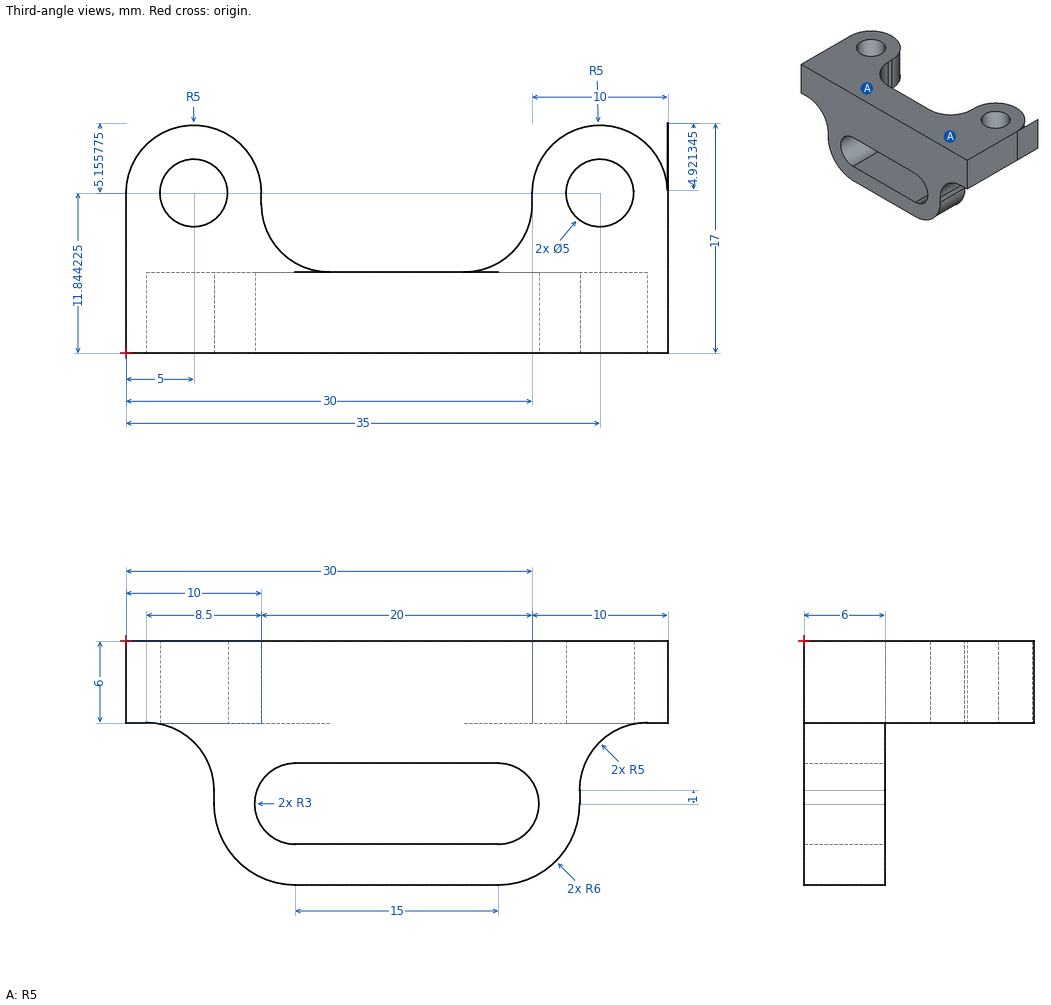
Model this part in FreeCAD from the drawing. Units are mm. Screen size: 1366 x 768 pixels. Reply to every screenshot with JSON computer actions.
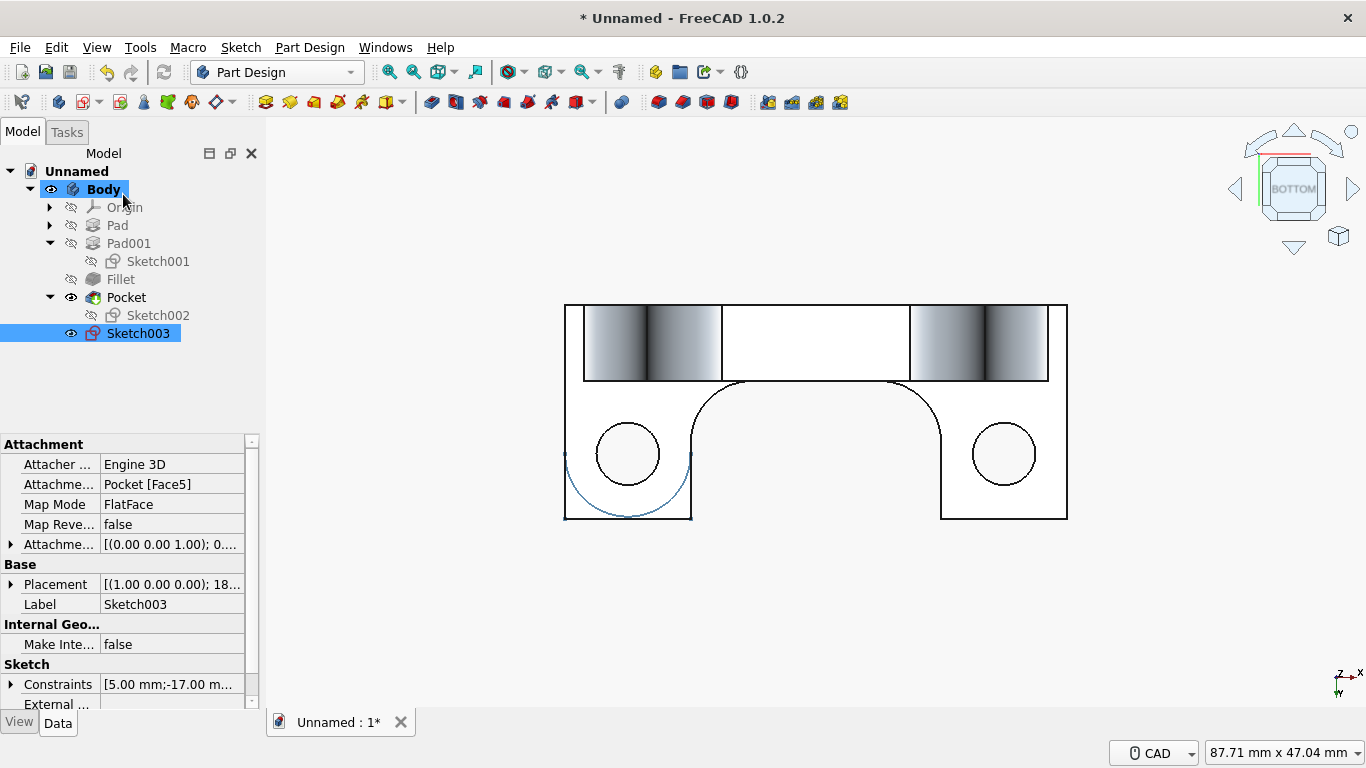
{"action": "left_click", "coordinate": [432, 102]}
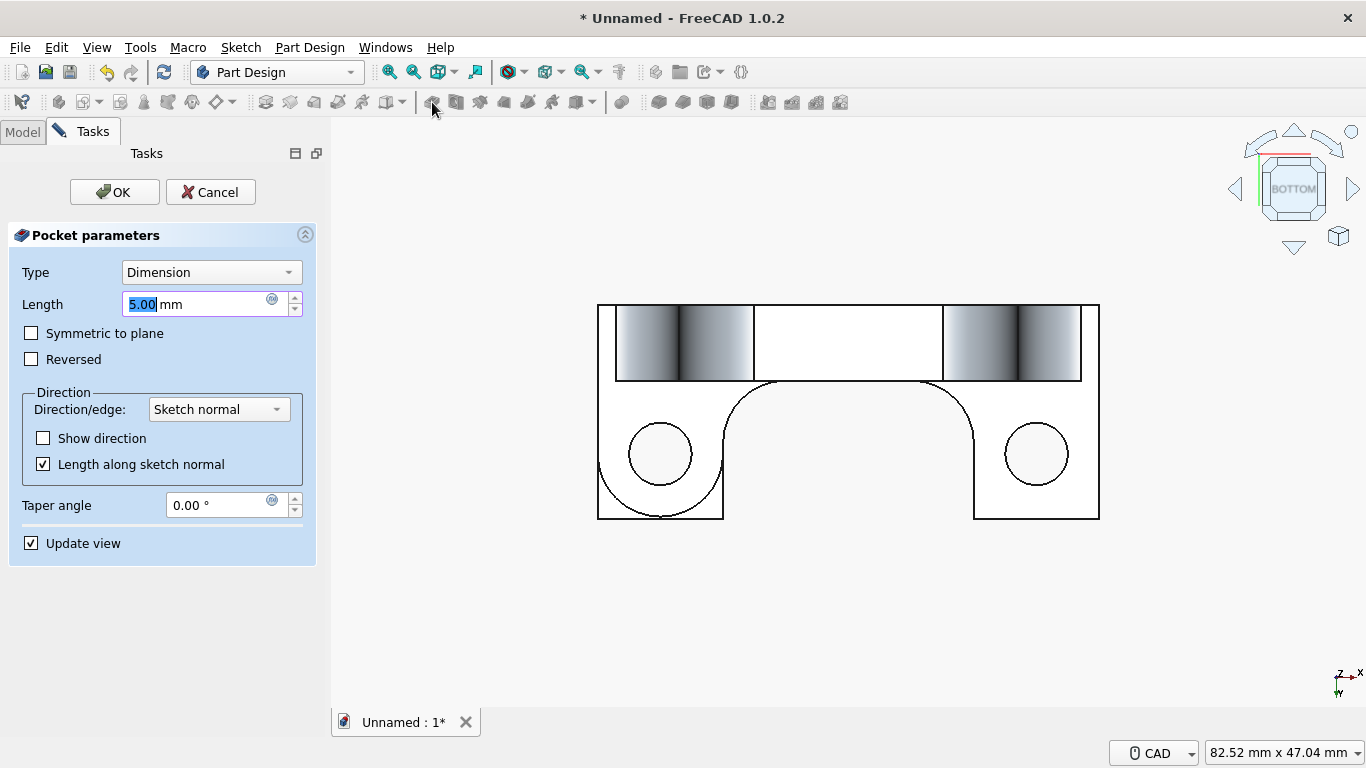
{"action": "type", "text": "17"}
{"action": "key", "text": "Tab"}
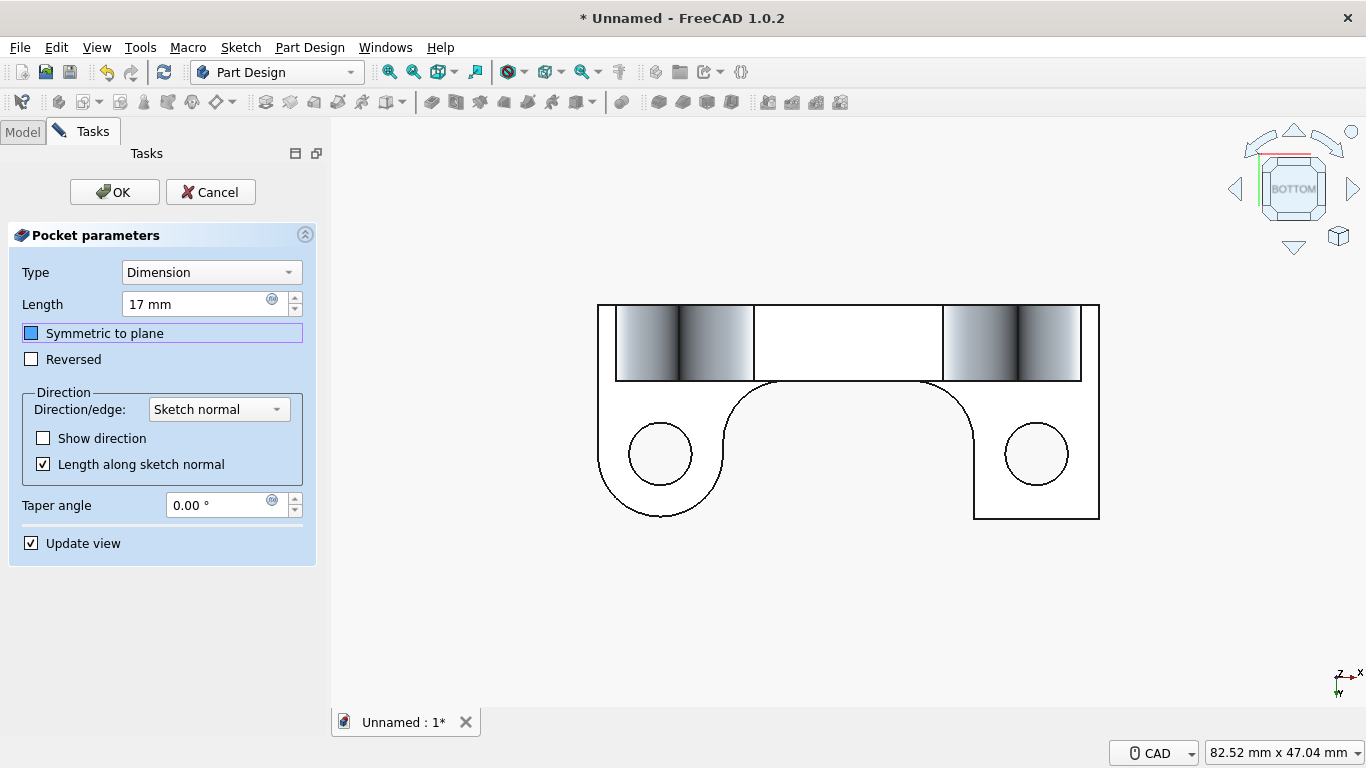
{"action": "left_click", "coordinate": [115, 192]}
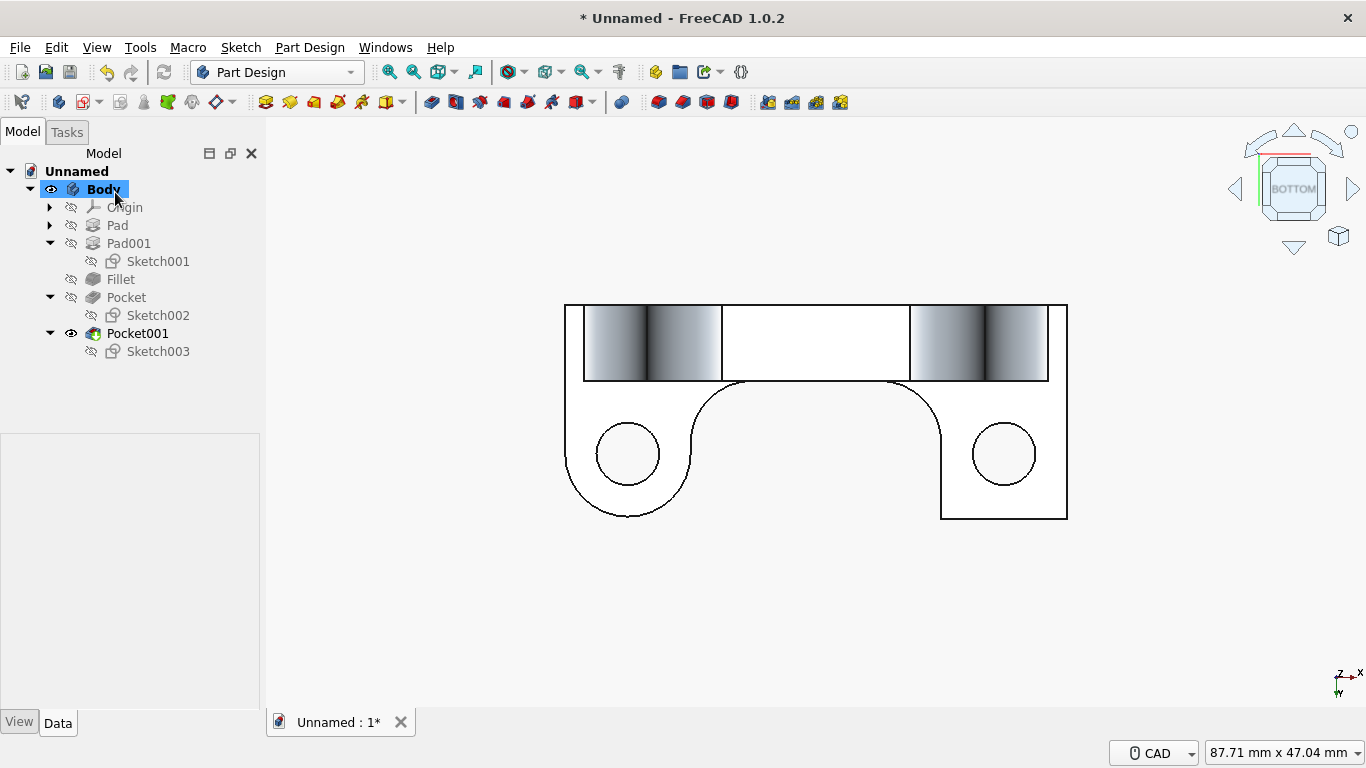
{"action": "left_click", "coordinate": [973, 411]}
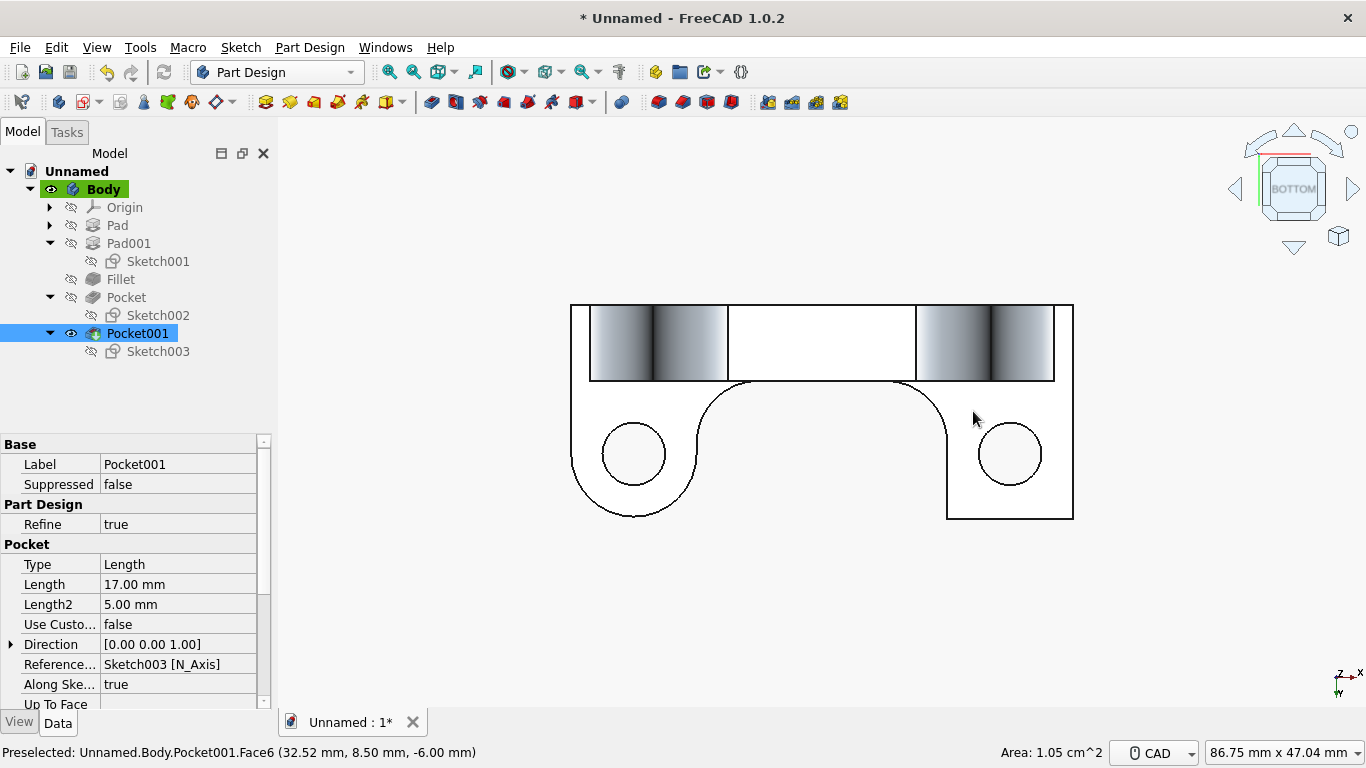
{"action": "left_click", "coordinate": [84, 102]}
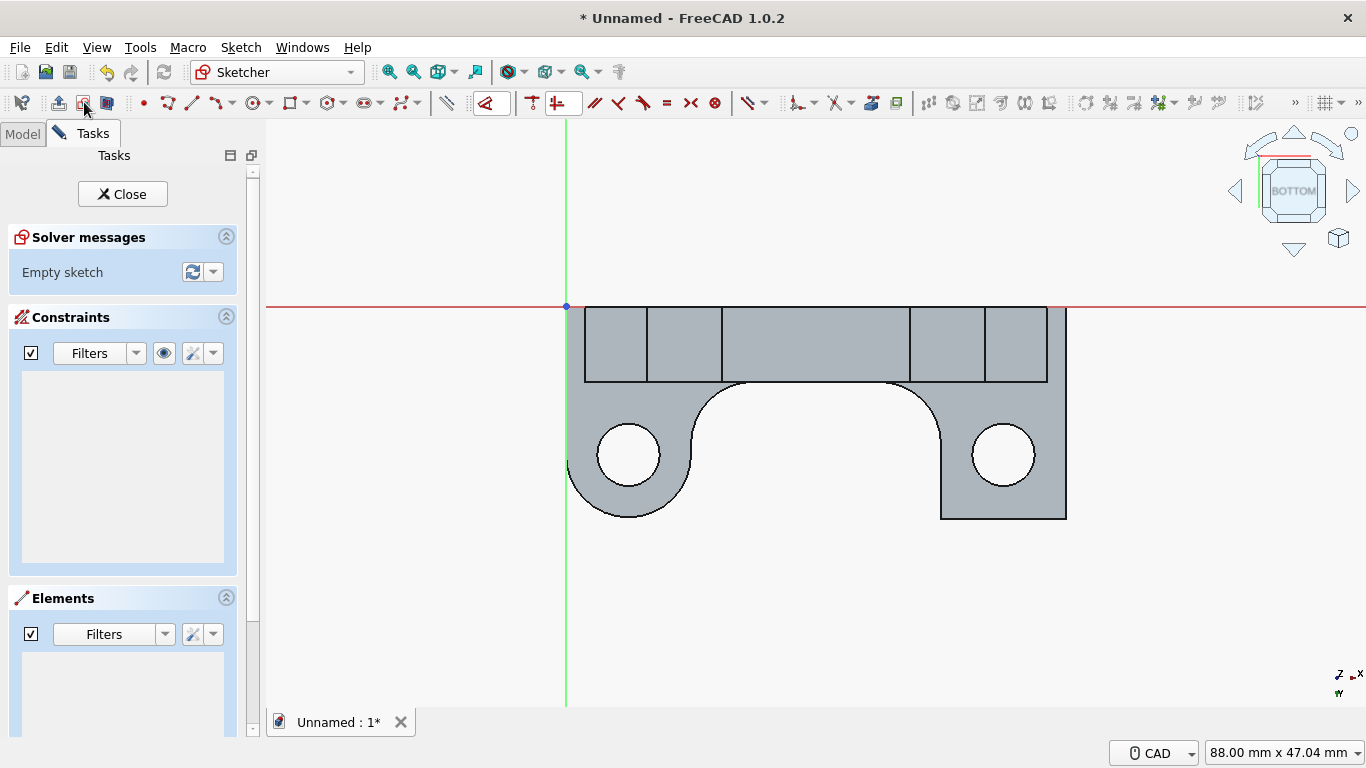
{"action": "key", "text": "q s"}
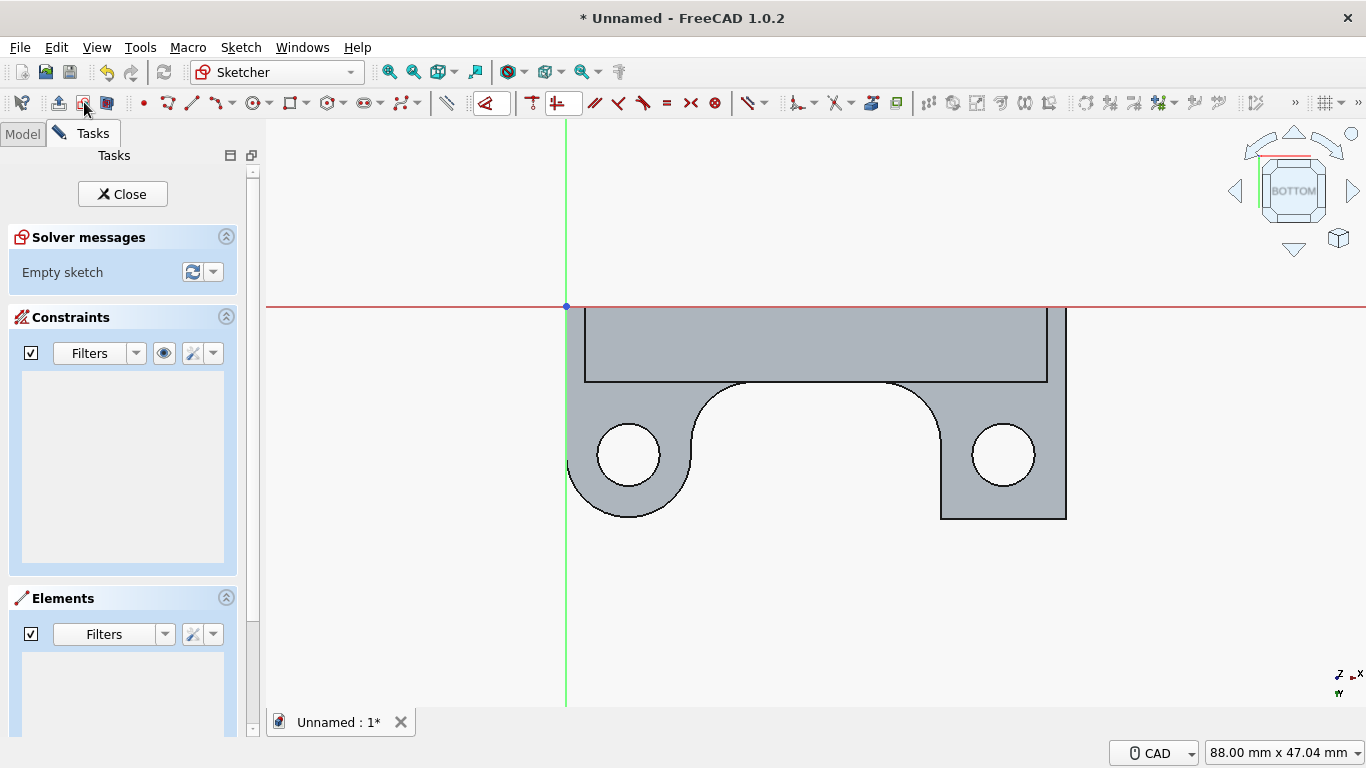
{"action": "scroll", "coordinate": [1068, 506], "scroll_direction": "up", "scroll_amount": 8}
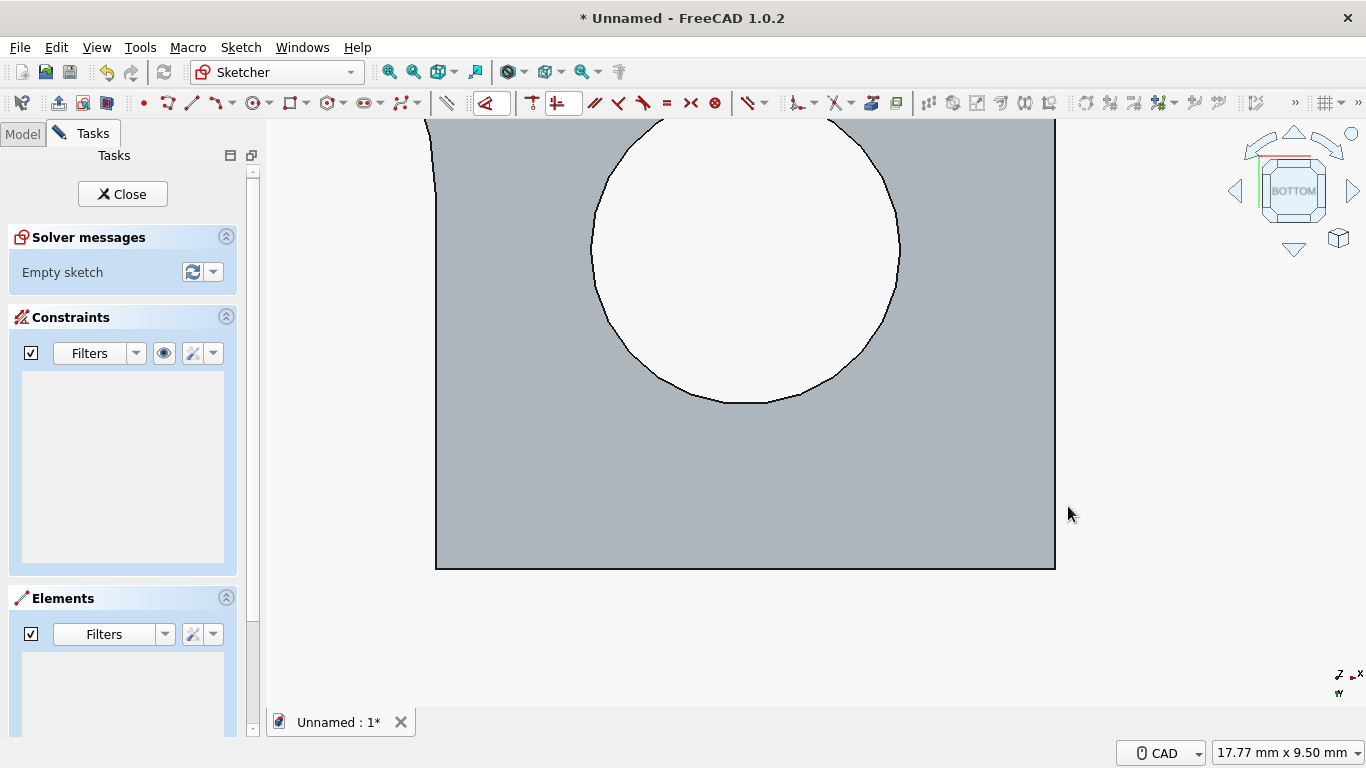
{"action": "key", "text": "g m"}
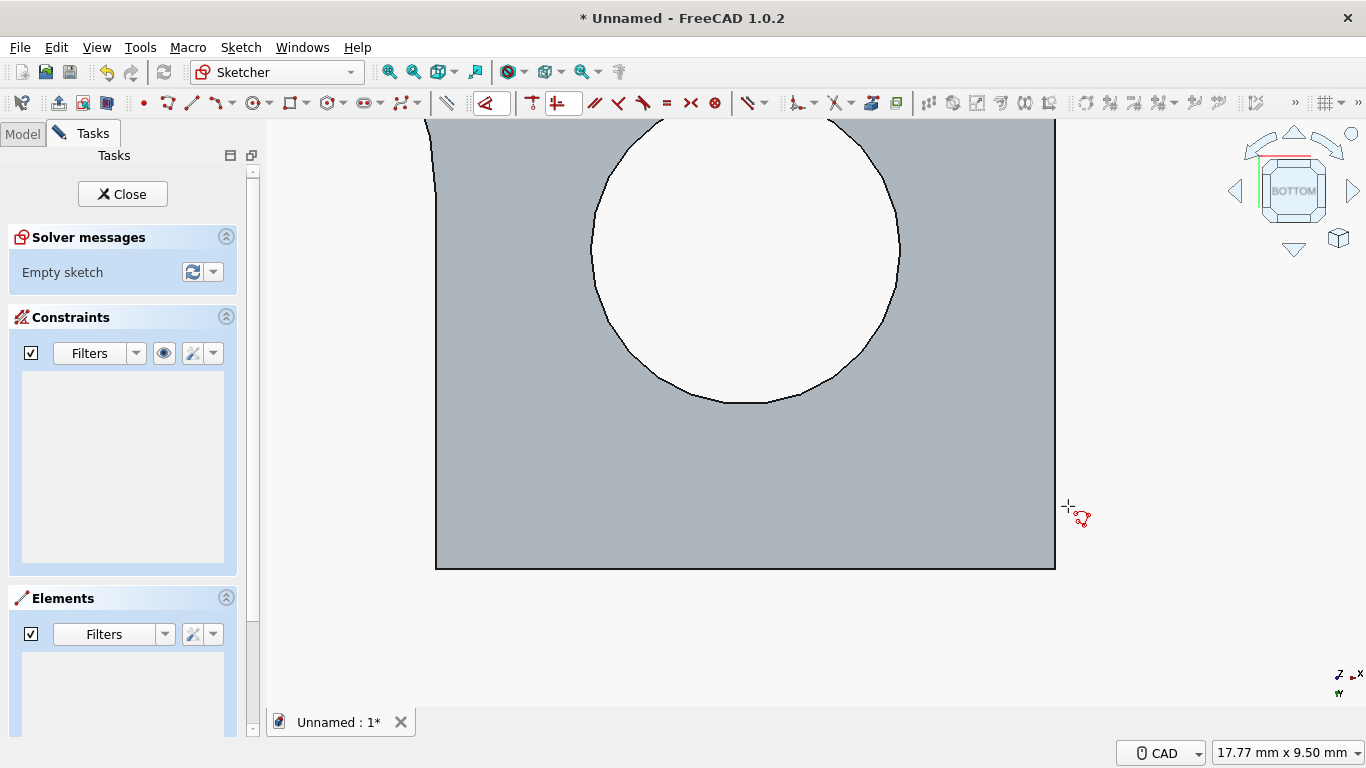
{"action": "left_click", "coordinate": [436, 250]}
{"action": "left_click", "coordinate": [436, 569]}
{"action": "left_click", "coordinate": [1055, 569]}
{"action": "left_click", "coordinate": [1040, 264]}
{"action": "right_click", "coordinate": [1040, 264]}